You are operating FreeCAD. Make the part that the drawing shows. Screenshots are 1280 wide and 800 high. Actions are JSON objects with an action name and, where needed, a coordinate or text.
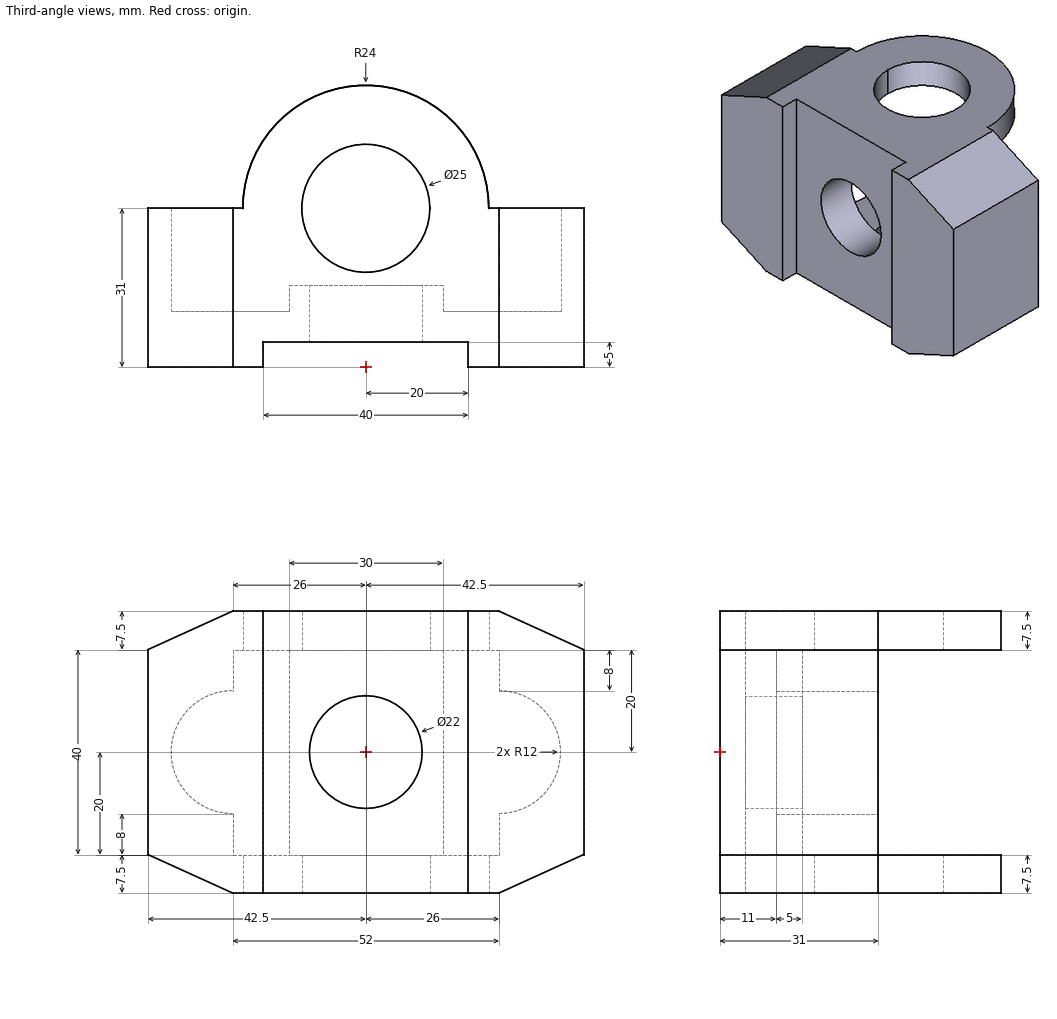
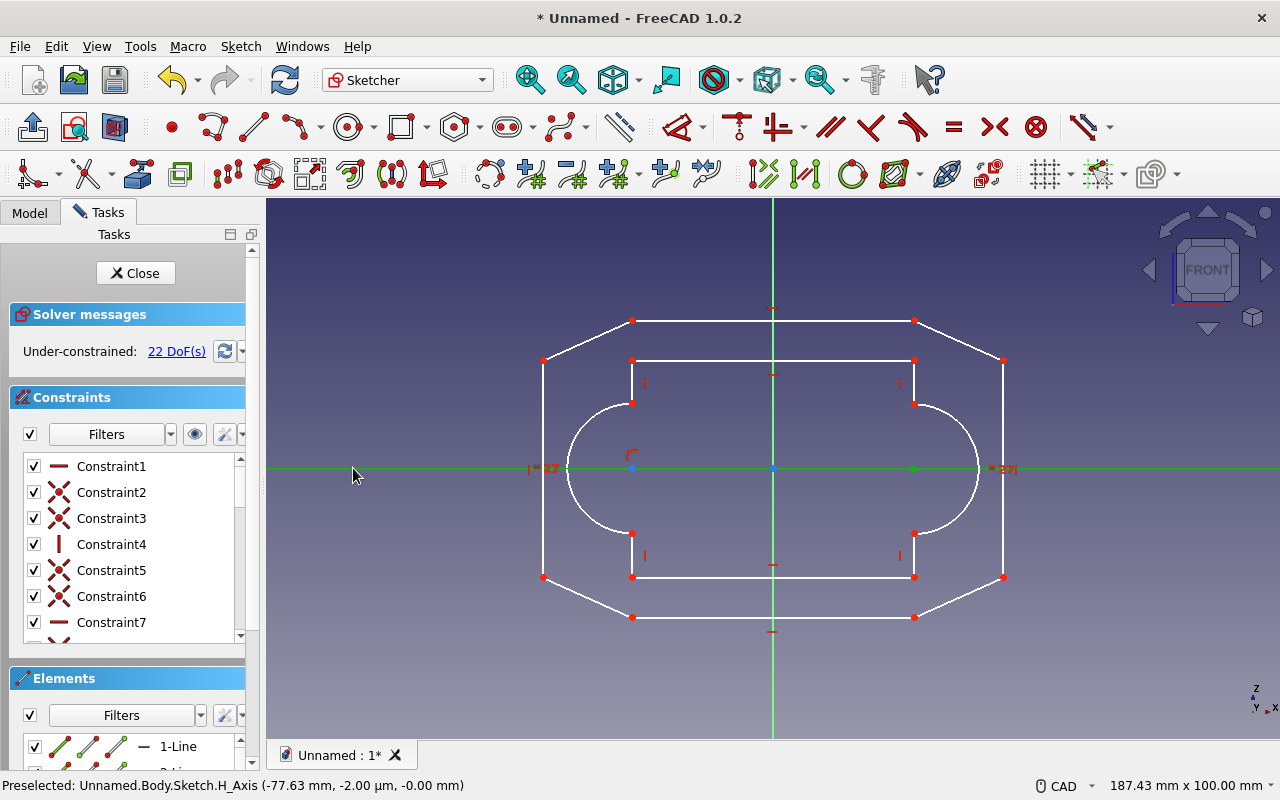
{"action": "key", "text": "c"}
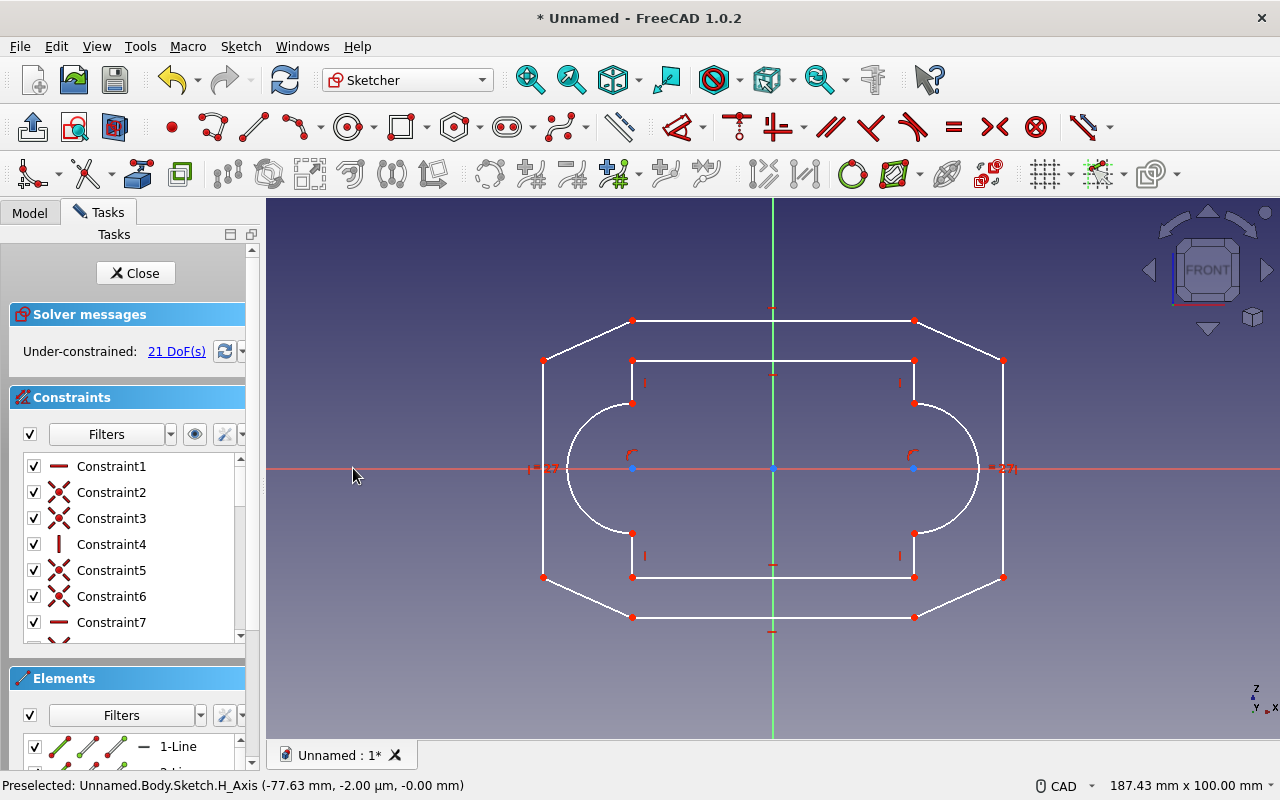
{"action": "left_click", "coordinate": [580, 430]}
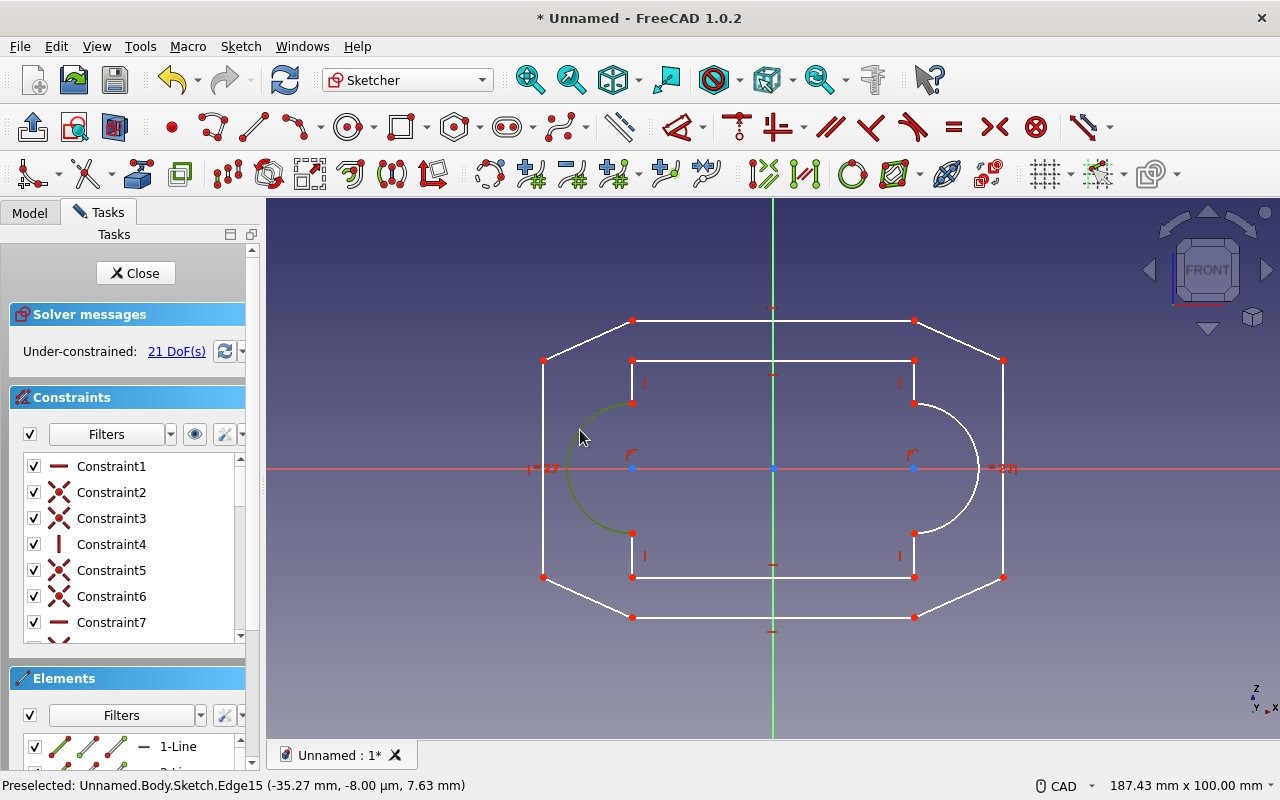
{"action": "left_click", "coordinate": [702, 128]}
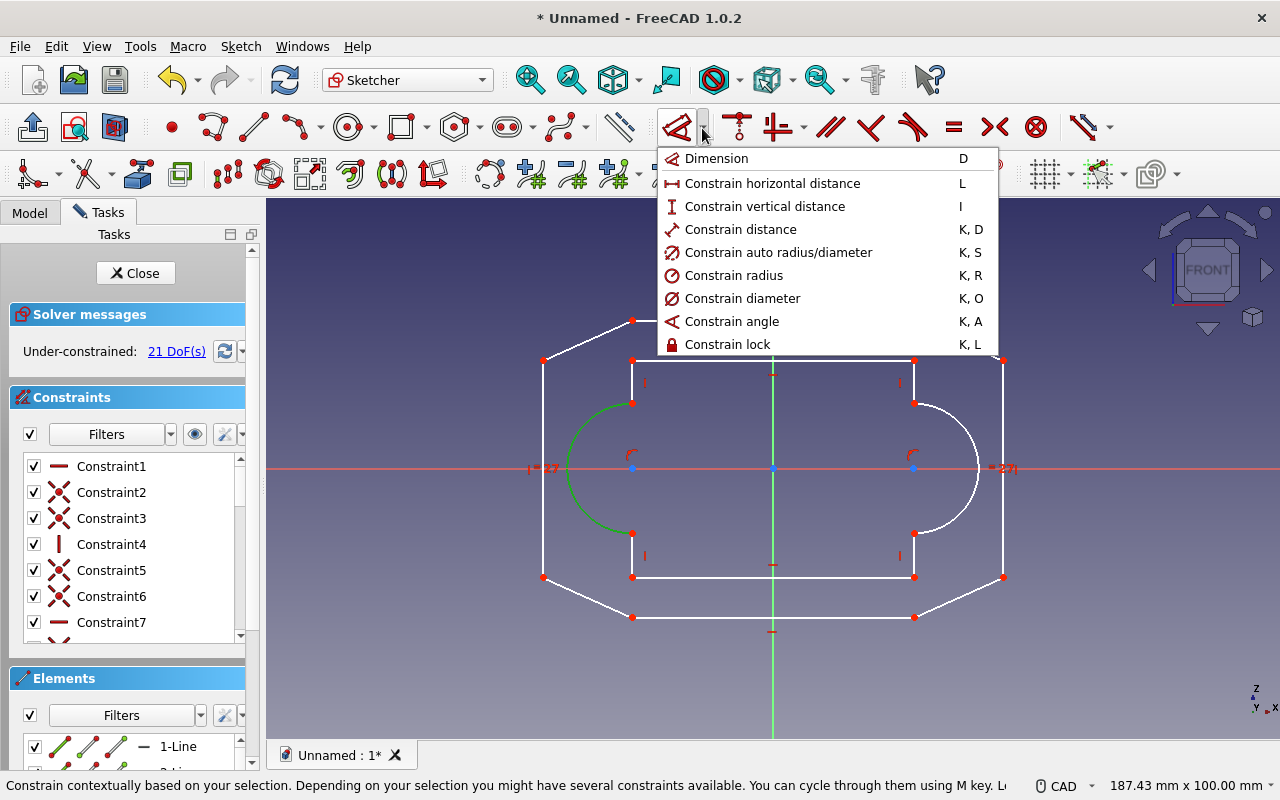
{"action": "left_click", "coordinate": [828, 276]}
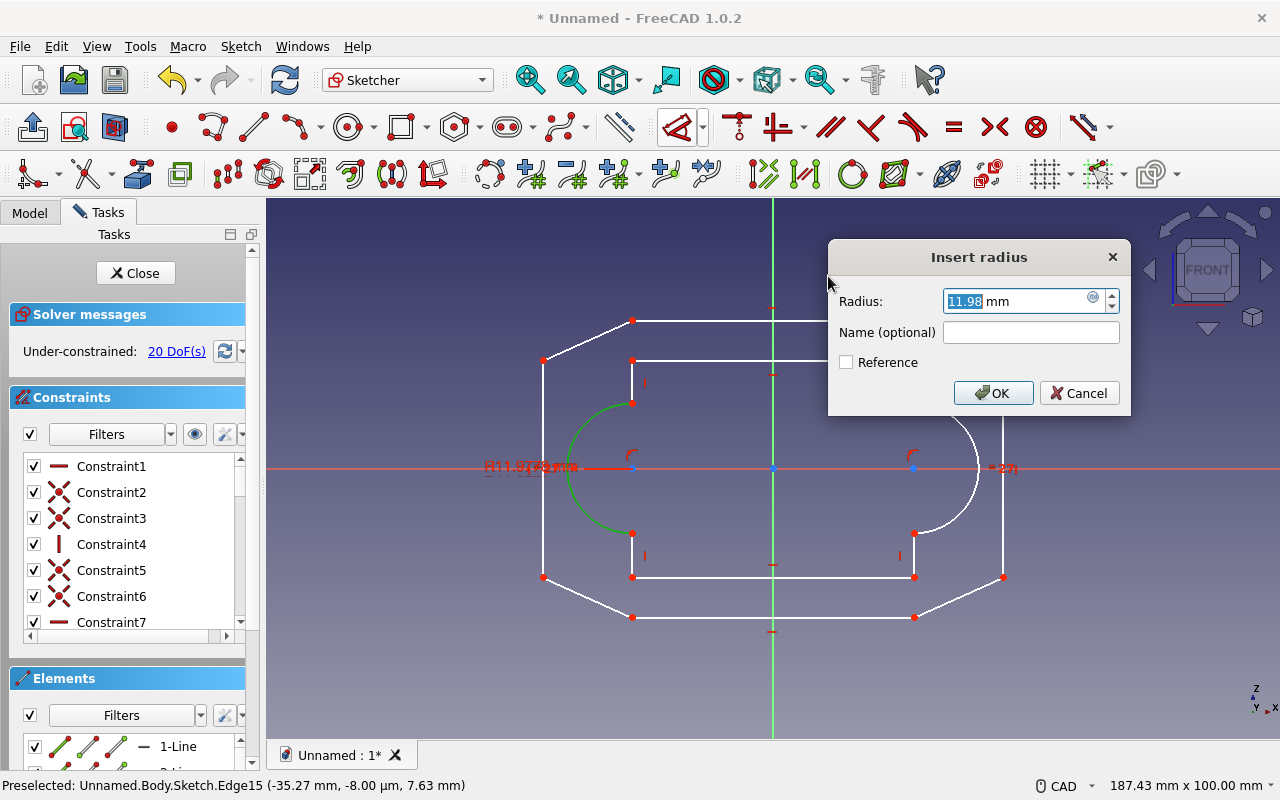
{"action": "type", "text": "12"}
{"action": "key", "text": "Return"}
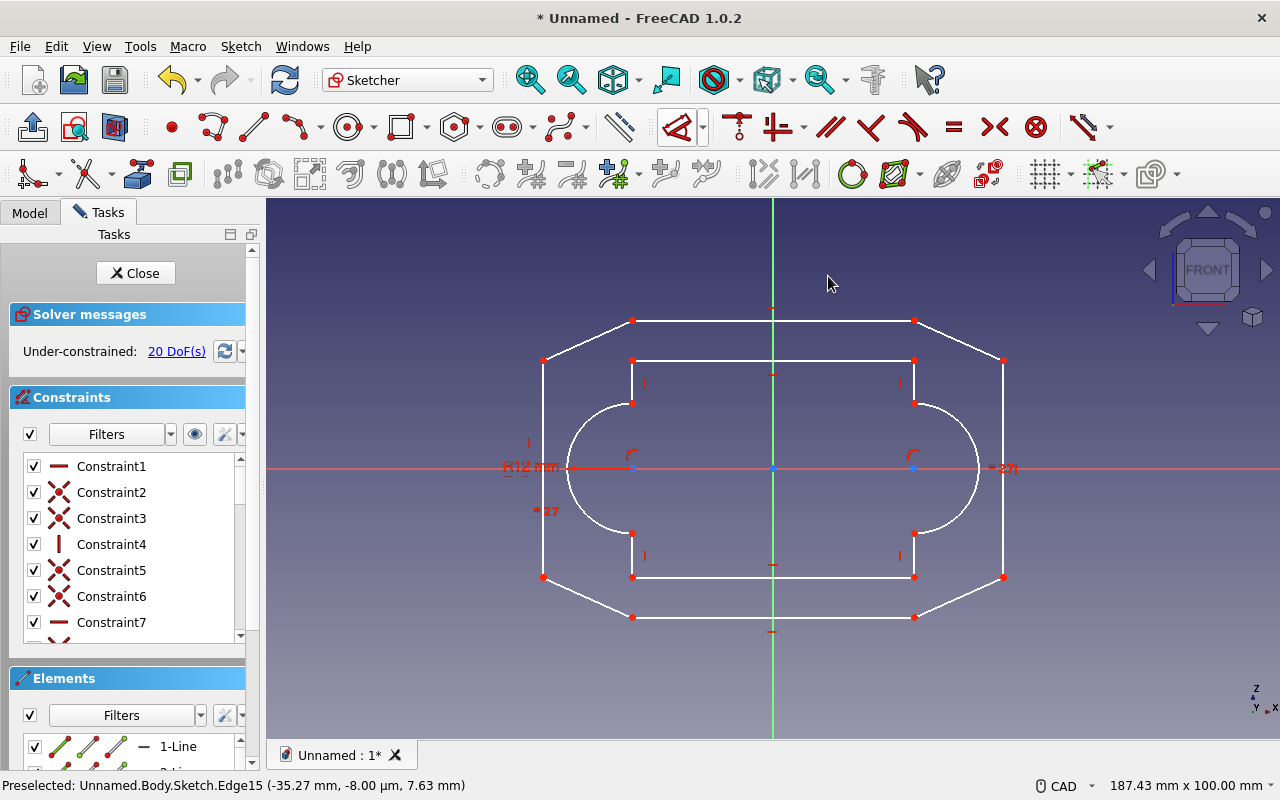
{"action": "left_click", "coordinate": [914, 391]}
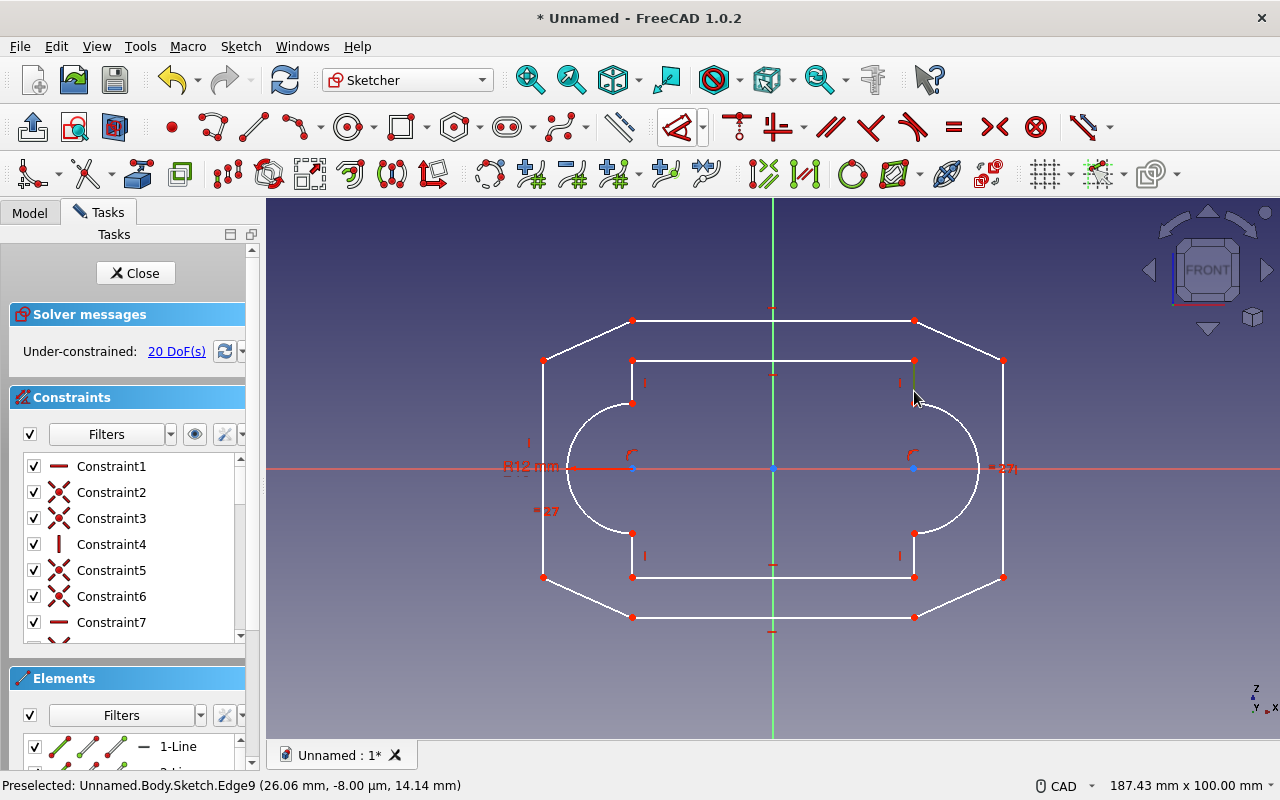
{"action": "key", "text": "i"}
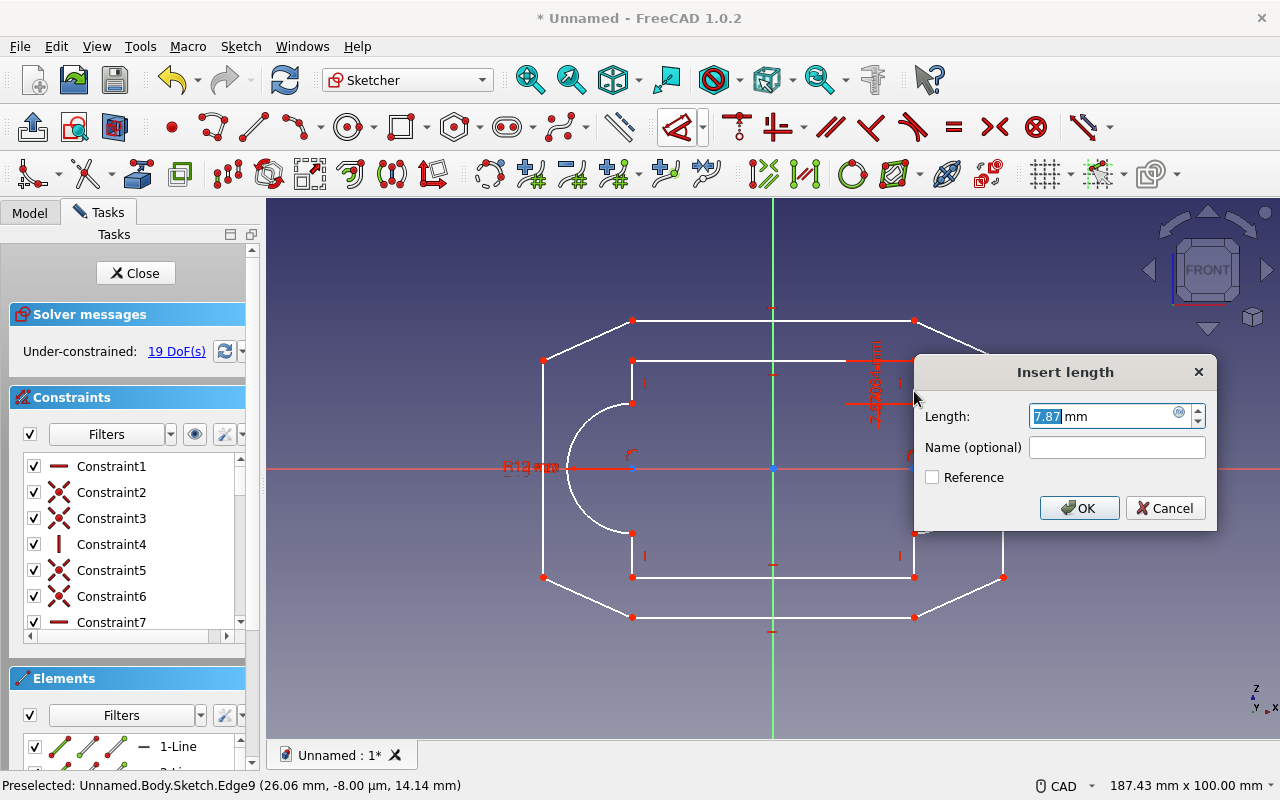
{"action": "type", "text": "8"}
{"action": "key", "text": "Return"}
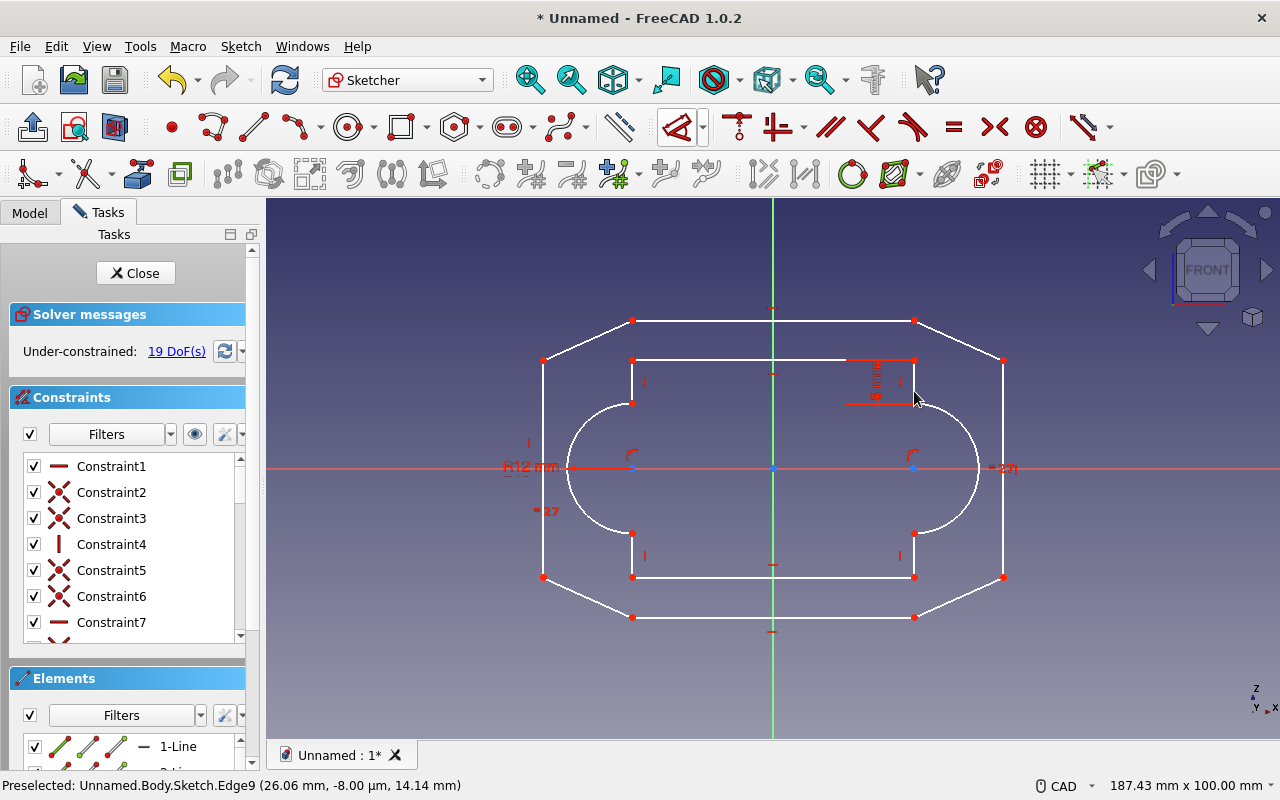
{"action": "left_click", "coordinate": [632, 547]}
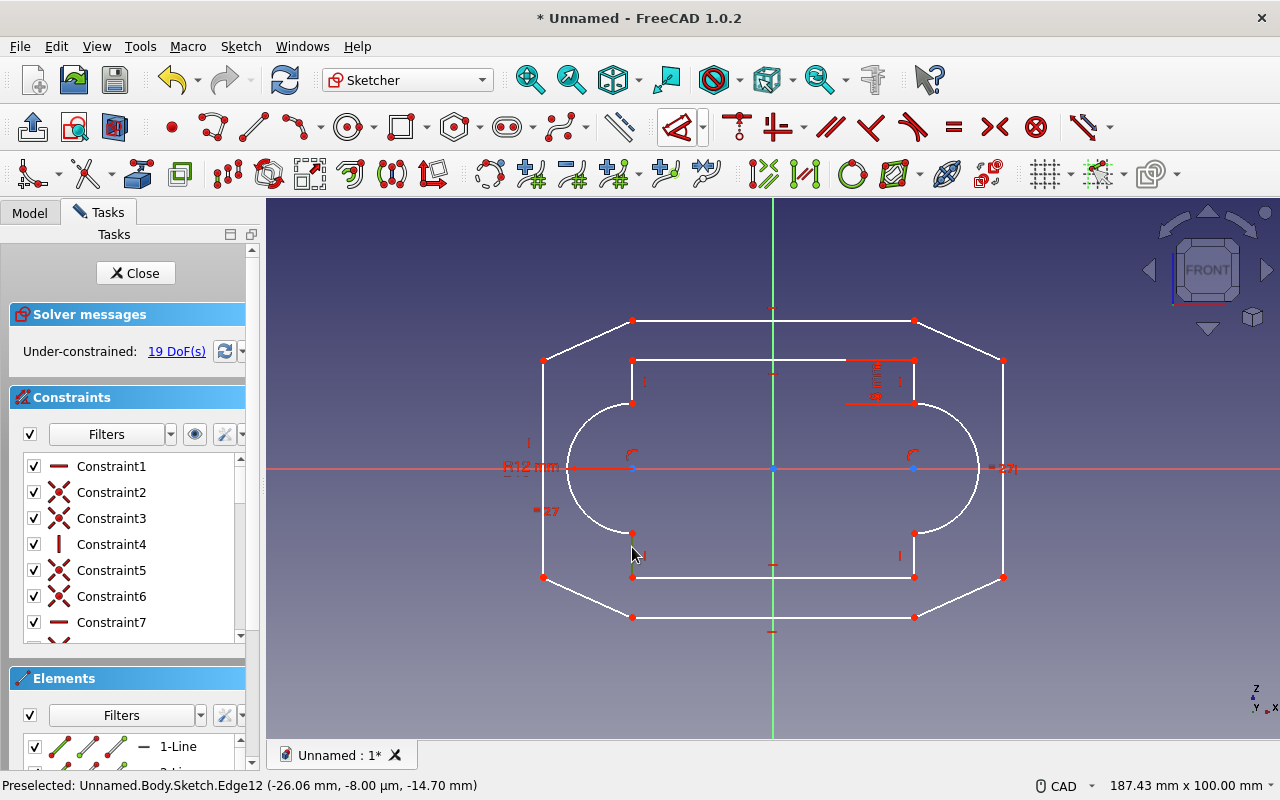
{"action": "key", "text": "i"}